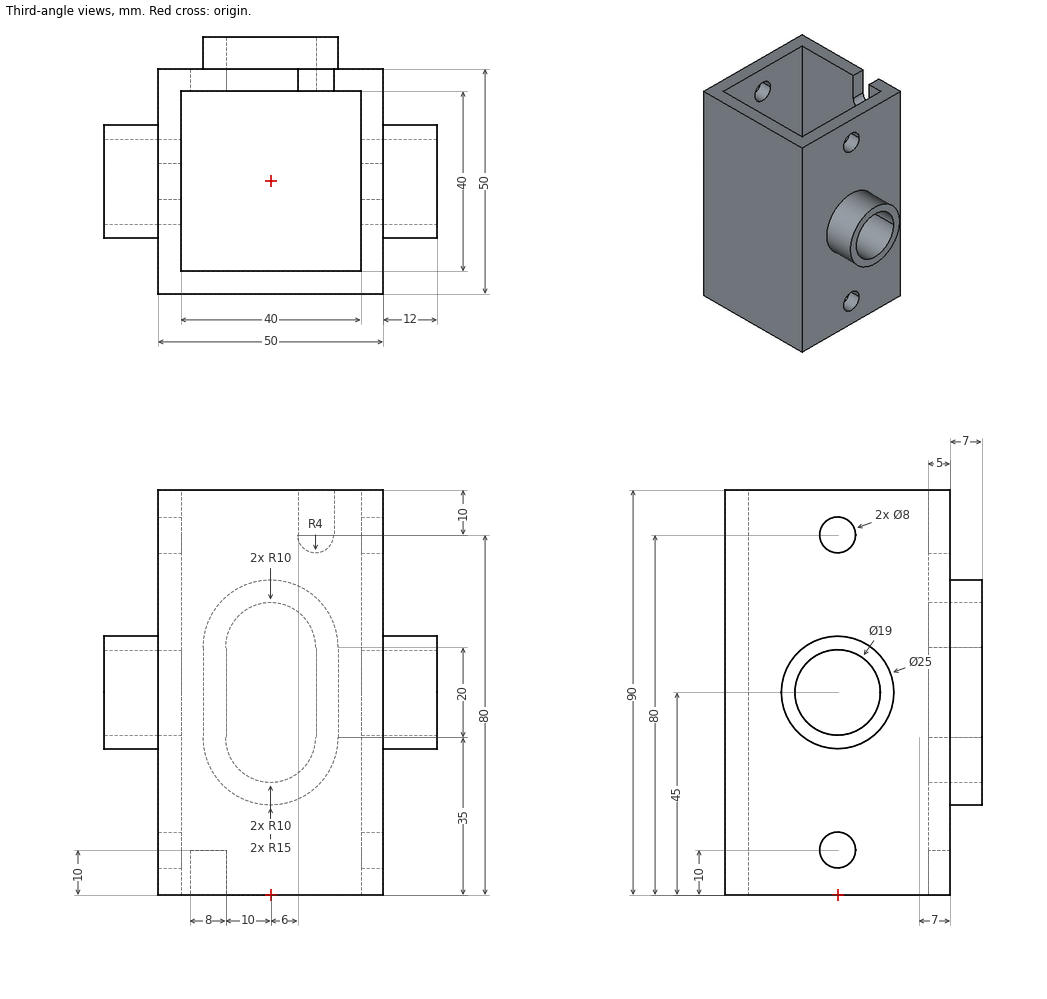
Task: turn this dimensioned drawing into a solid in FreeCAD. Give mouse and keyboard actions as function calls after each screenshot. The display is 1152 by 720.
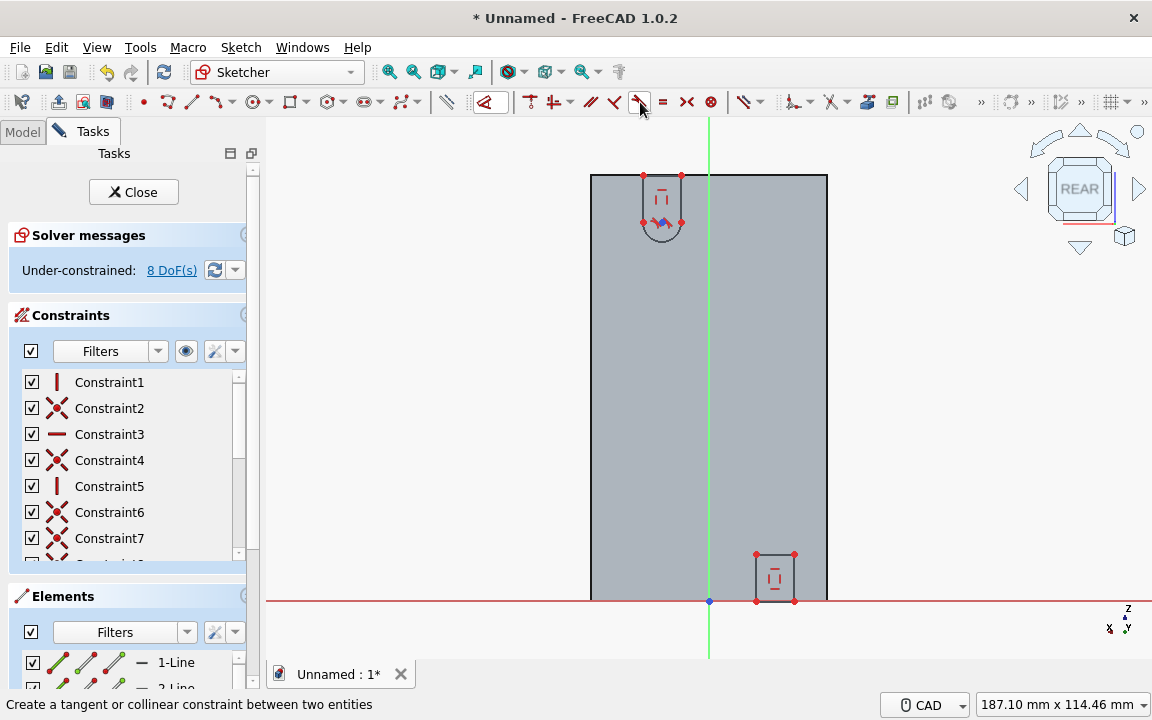
key(d)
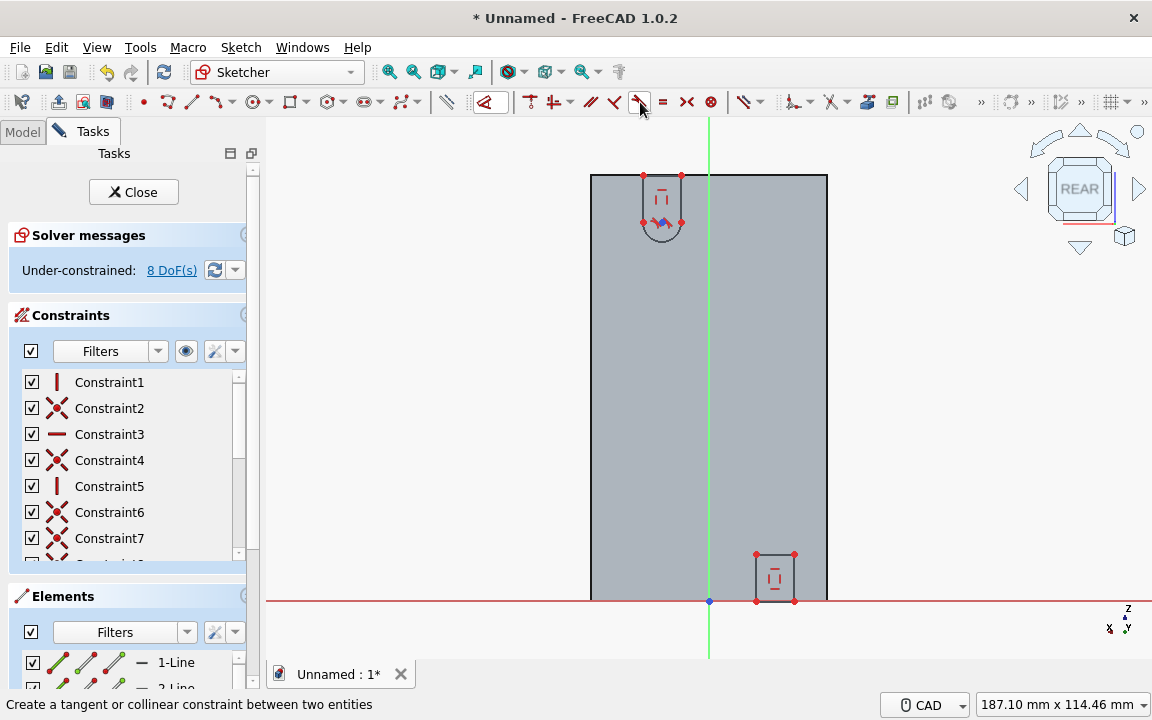
scroll(651, 238, up, 4)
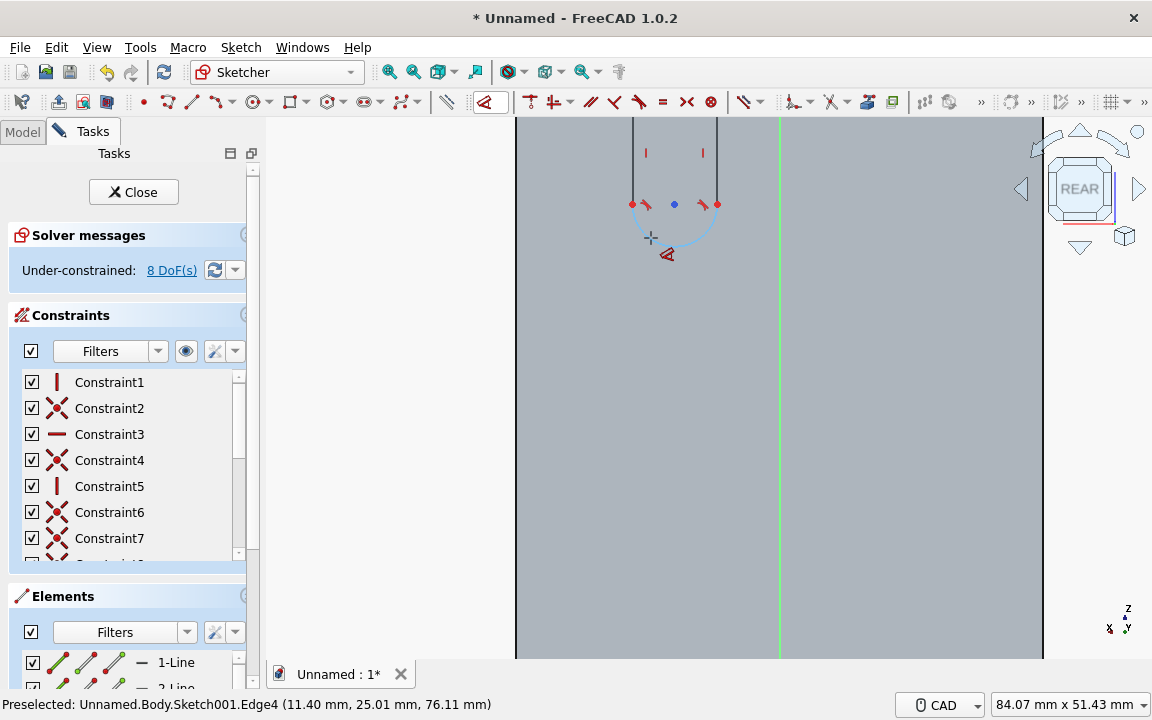
click(650, 239)
click(631, 265)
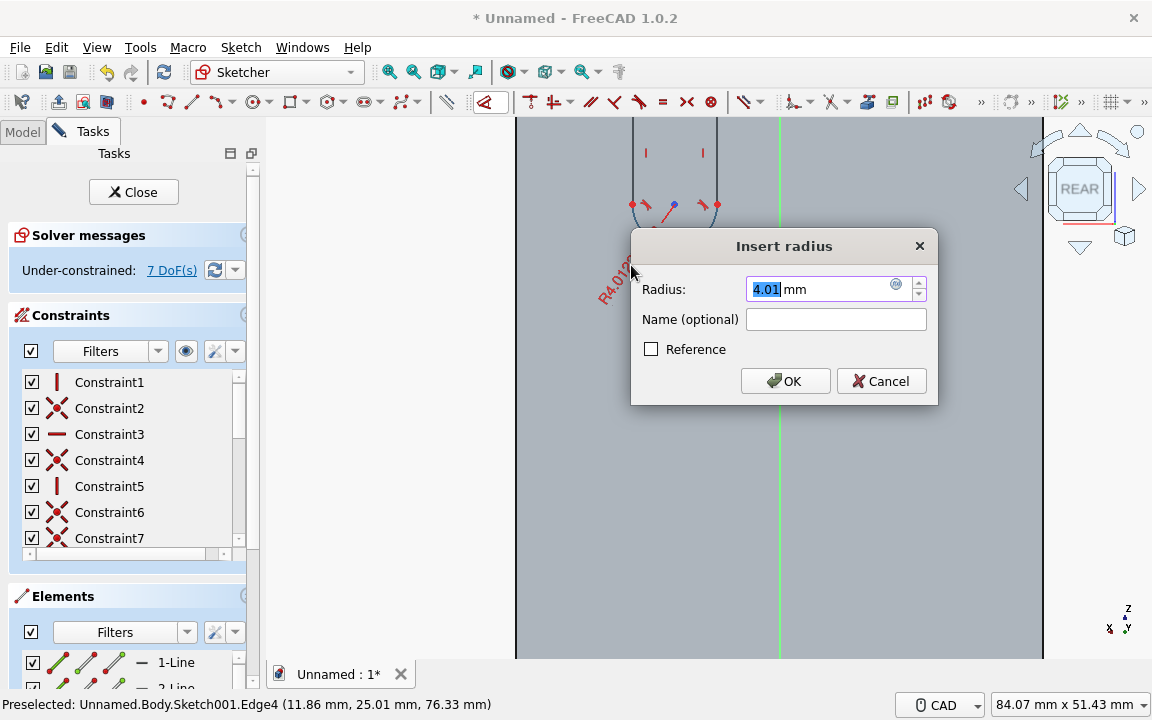
text(4)
key(Return)
key(Escape)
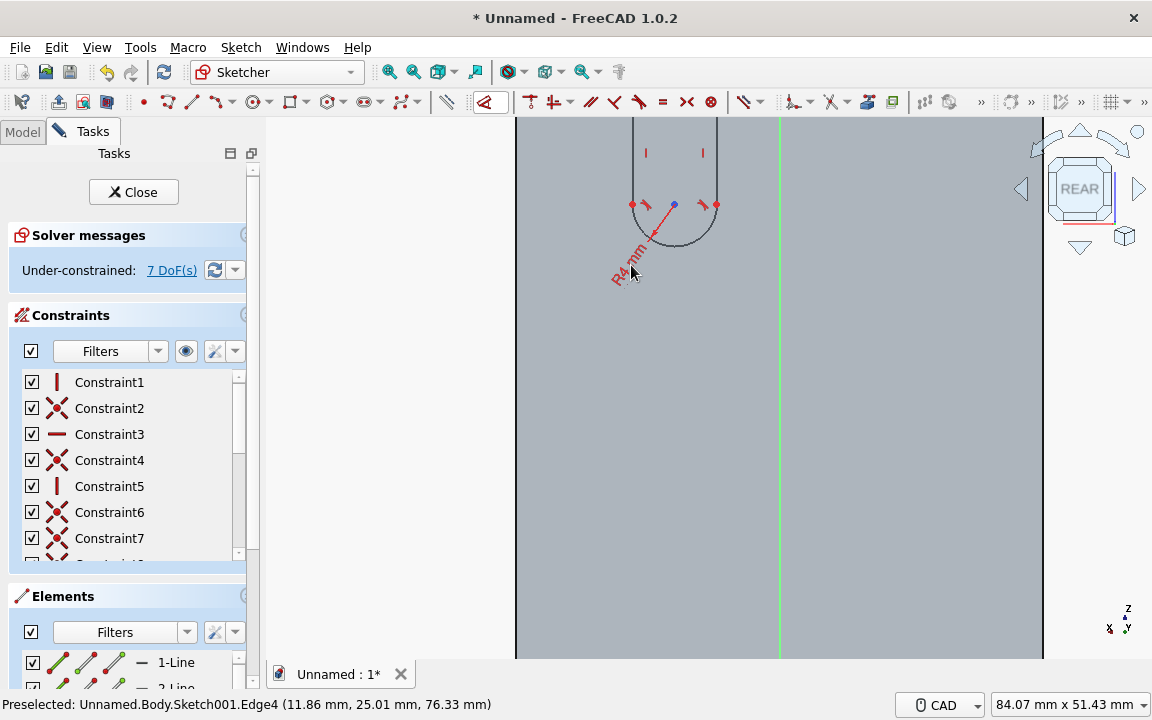
scroll(547, 281, down, 5)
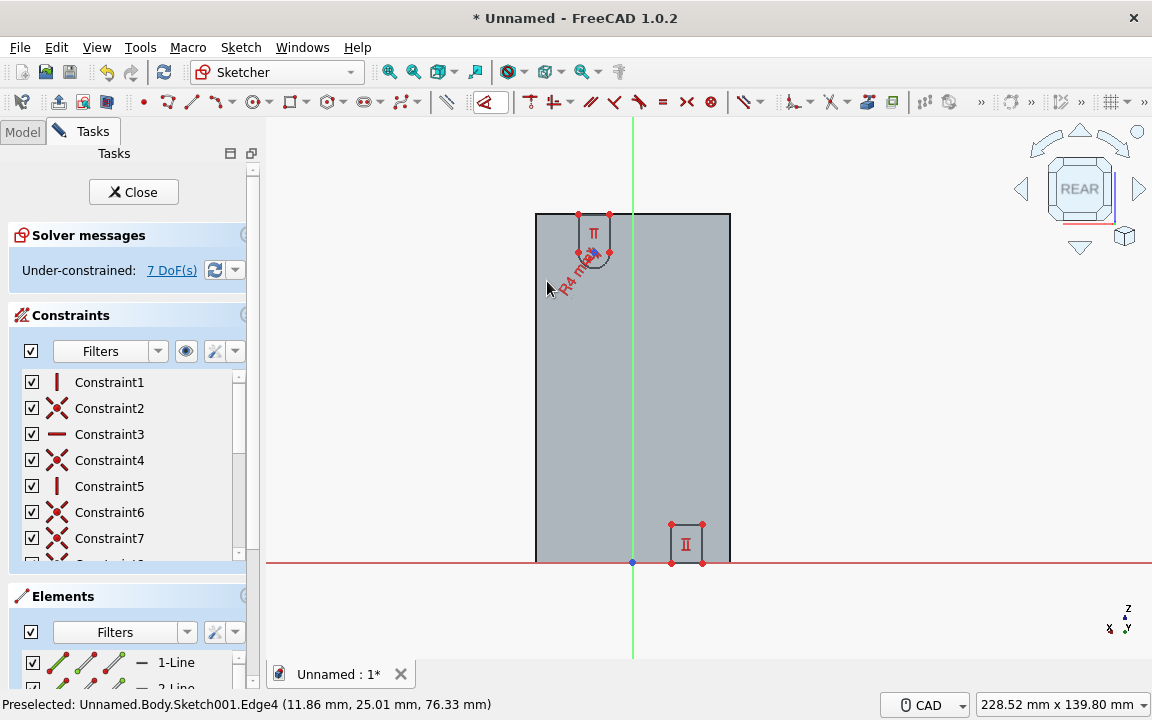
click(671, 563)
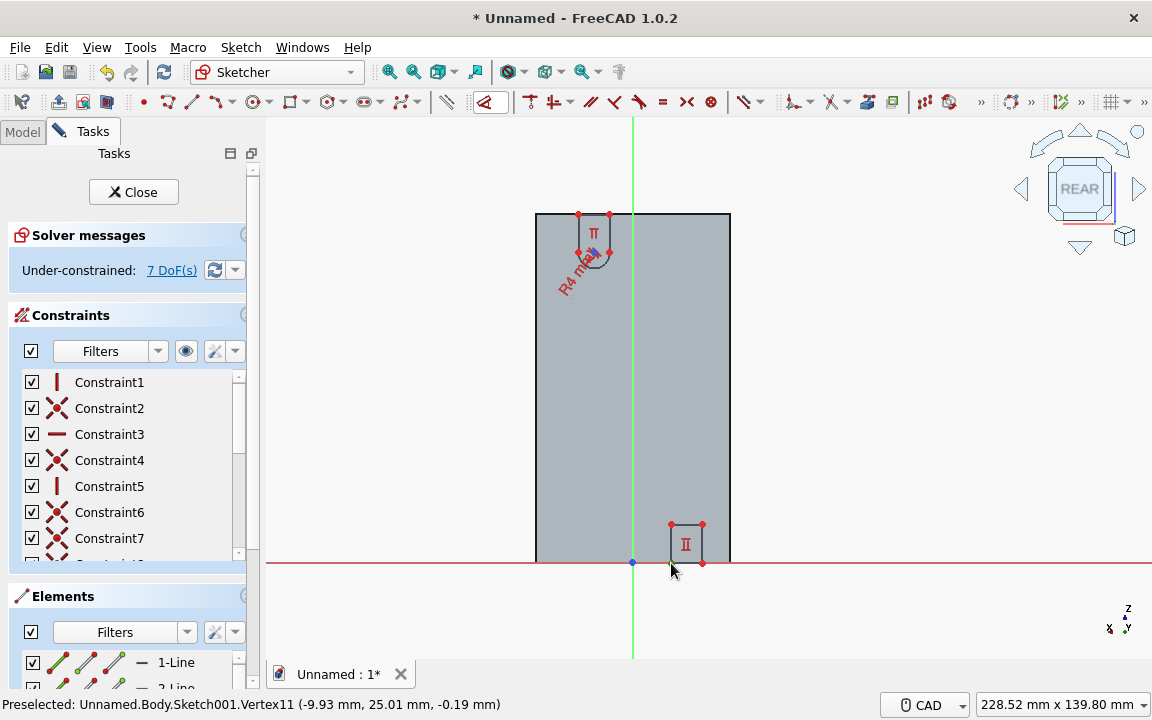
click(343, 563)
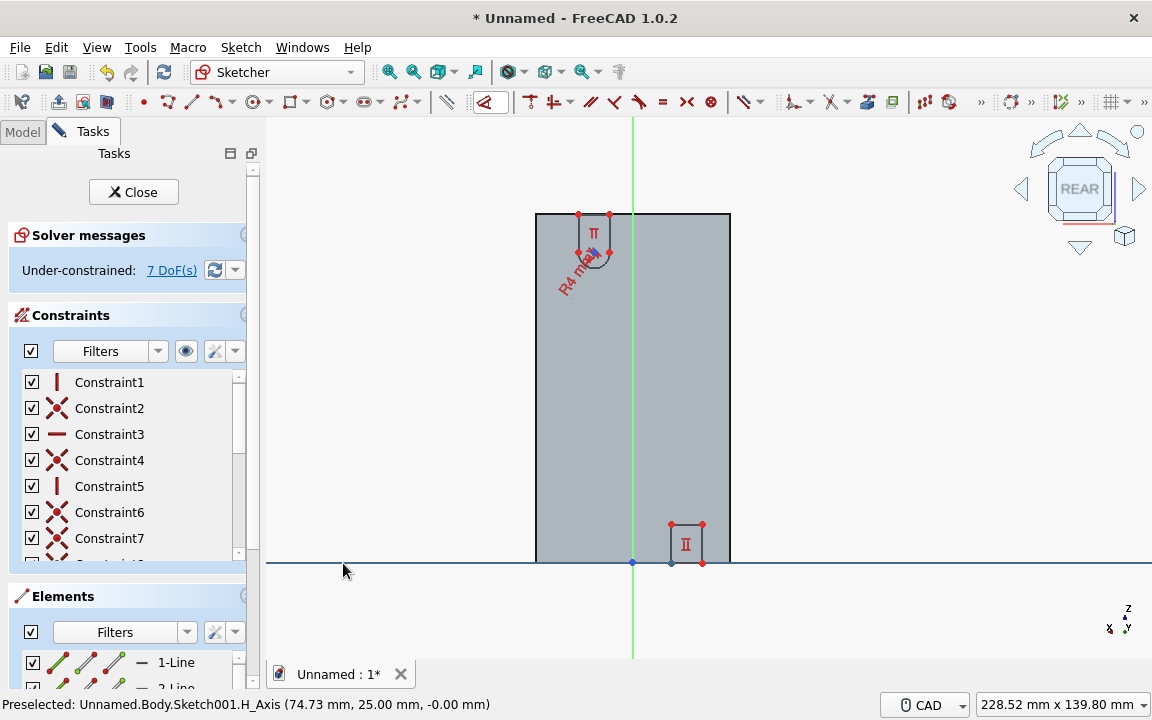
key(c)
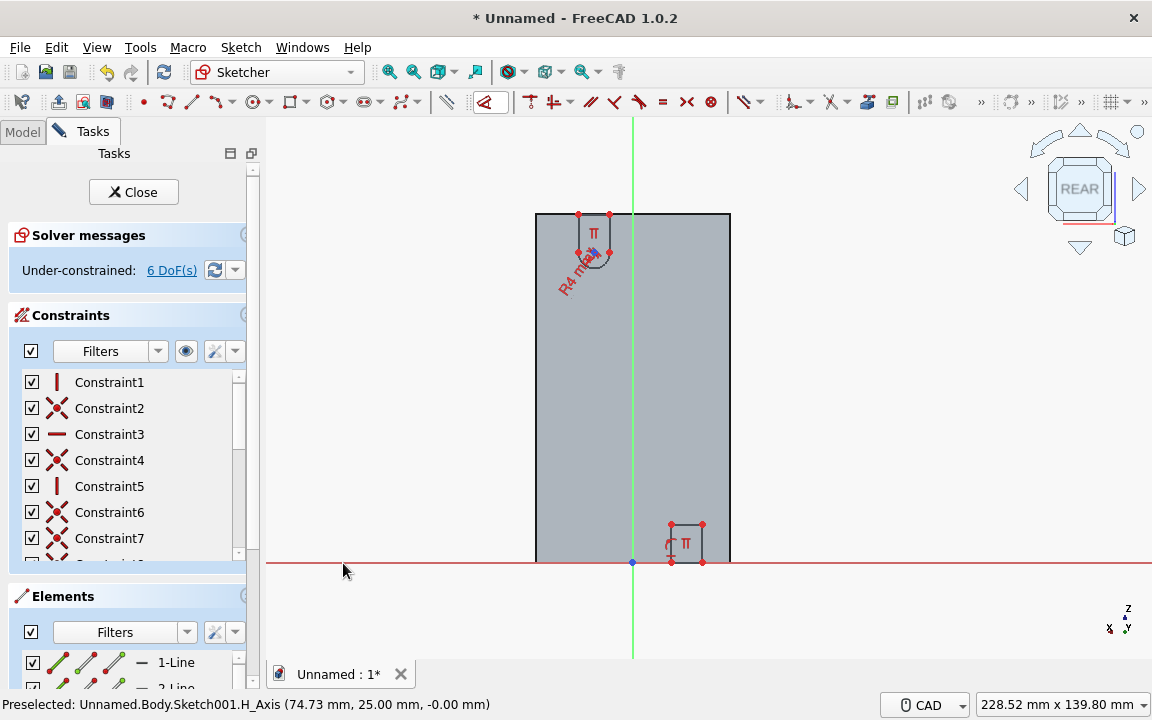
key(d)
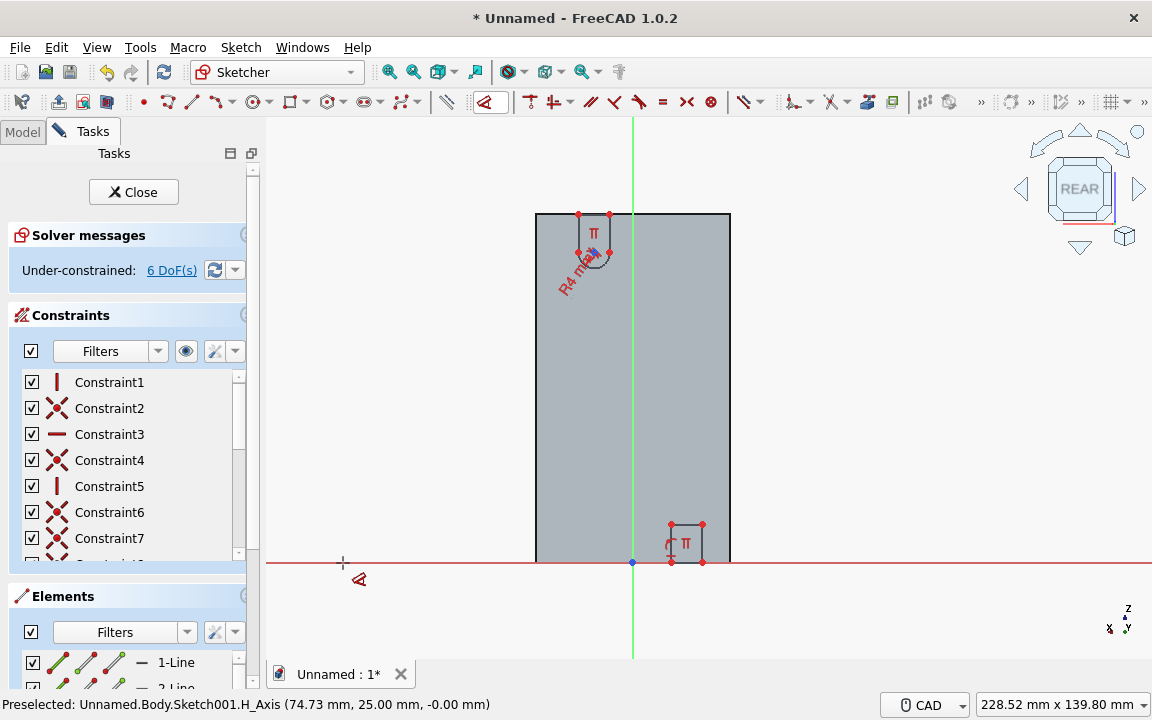
scroll(681, 563, up, 2)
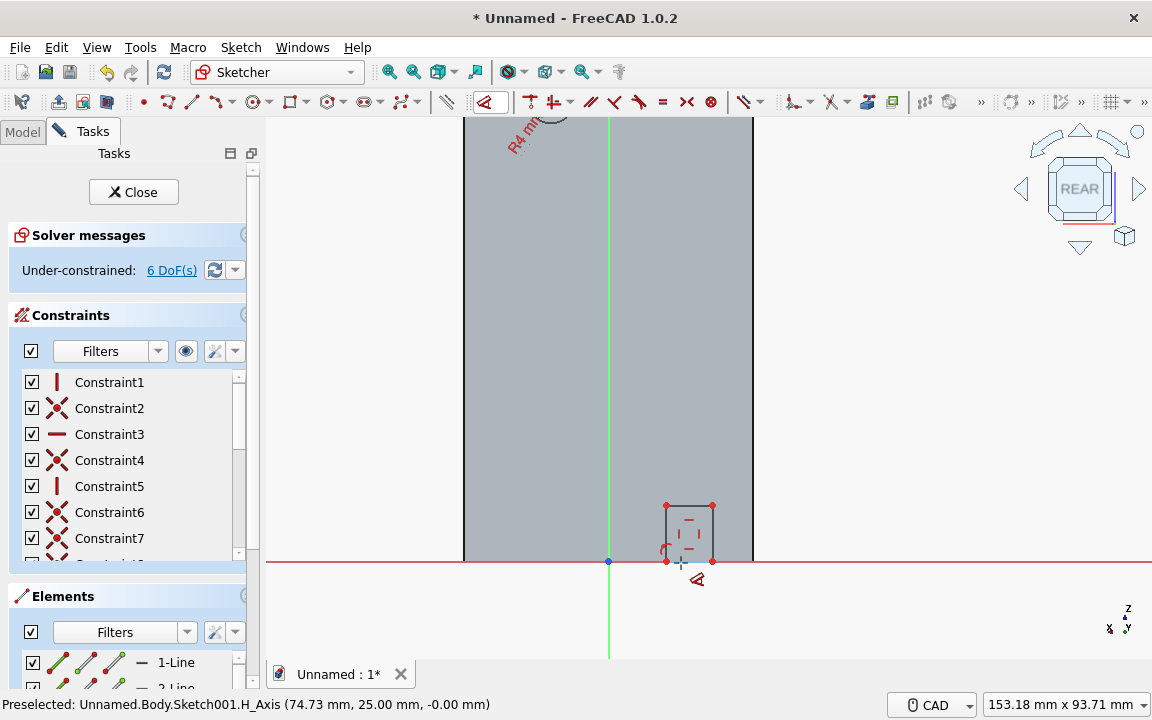
click(680, 562)
click(689, 596)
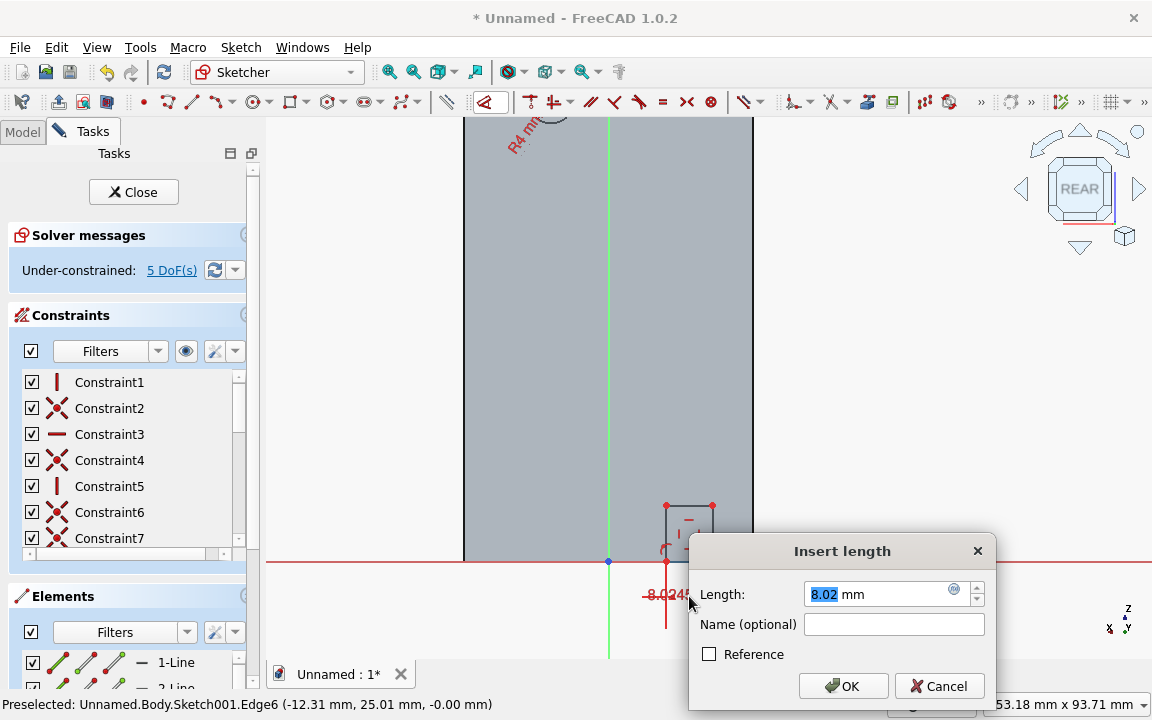
text(8)
key(Return)